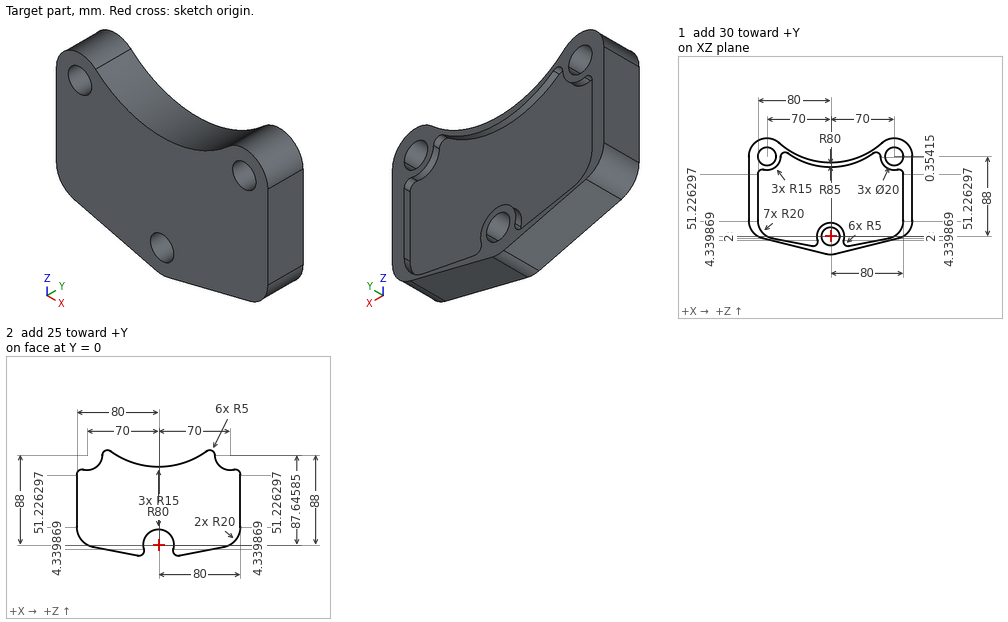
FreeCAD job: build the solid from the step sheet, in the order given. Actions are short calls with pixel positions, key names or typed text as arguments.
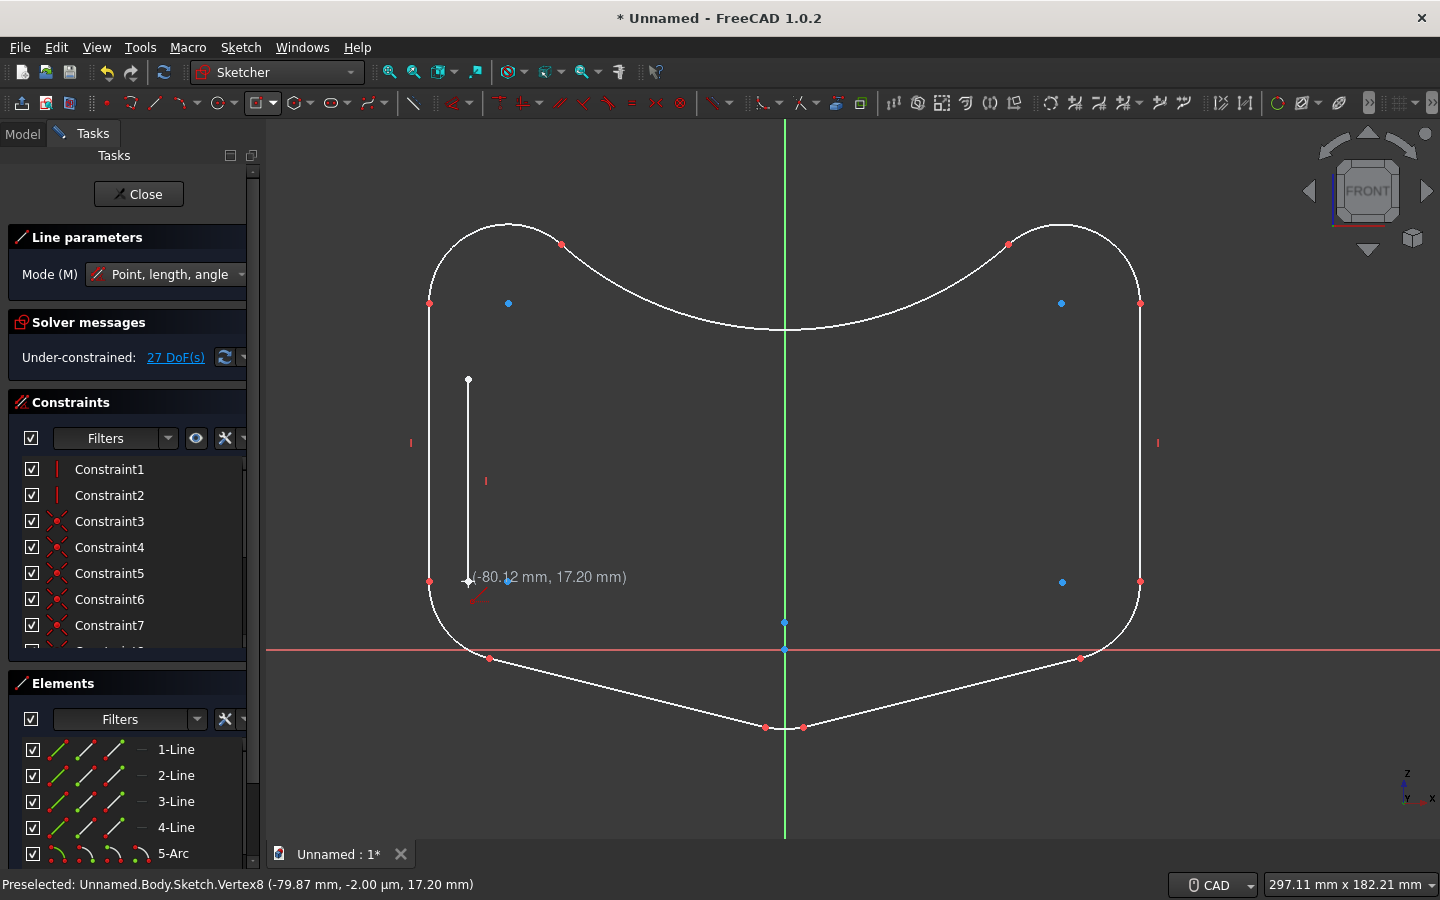
scroll(532, 659, up, 3)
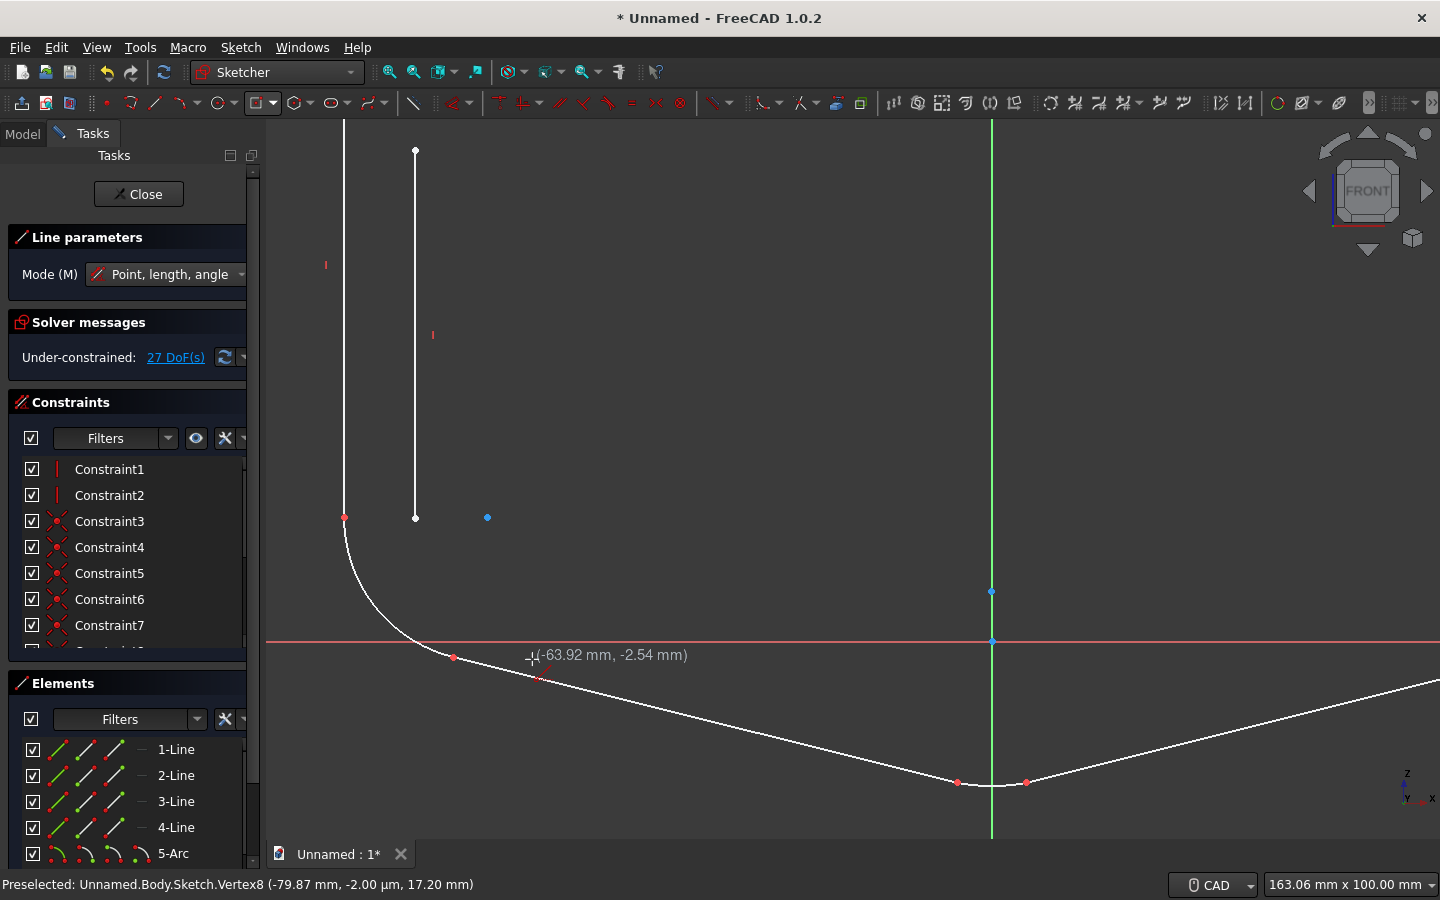
click(533, 658)
click(847, 719)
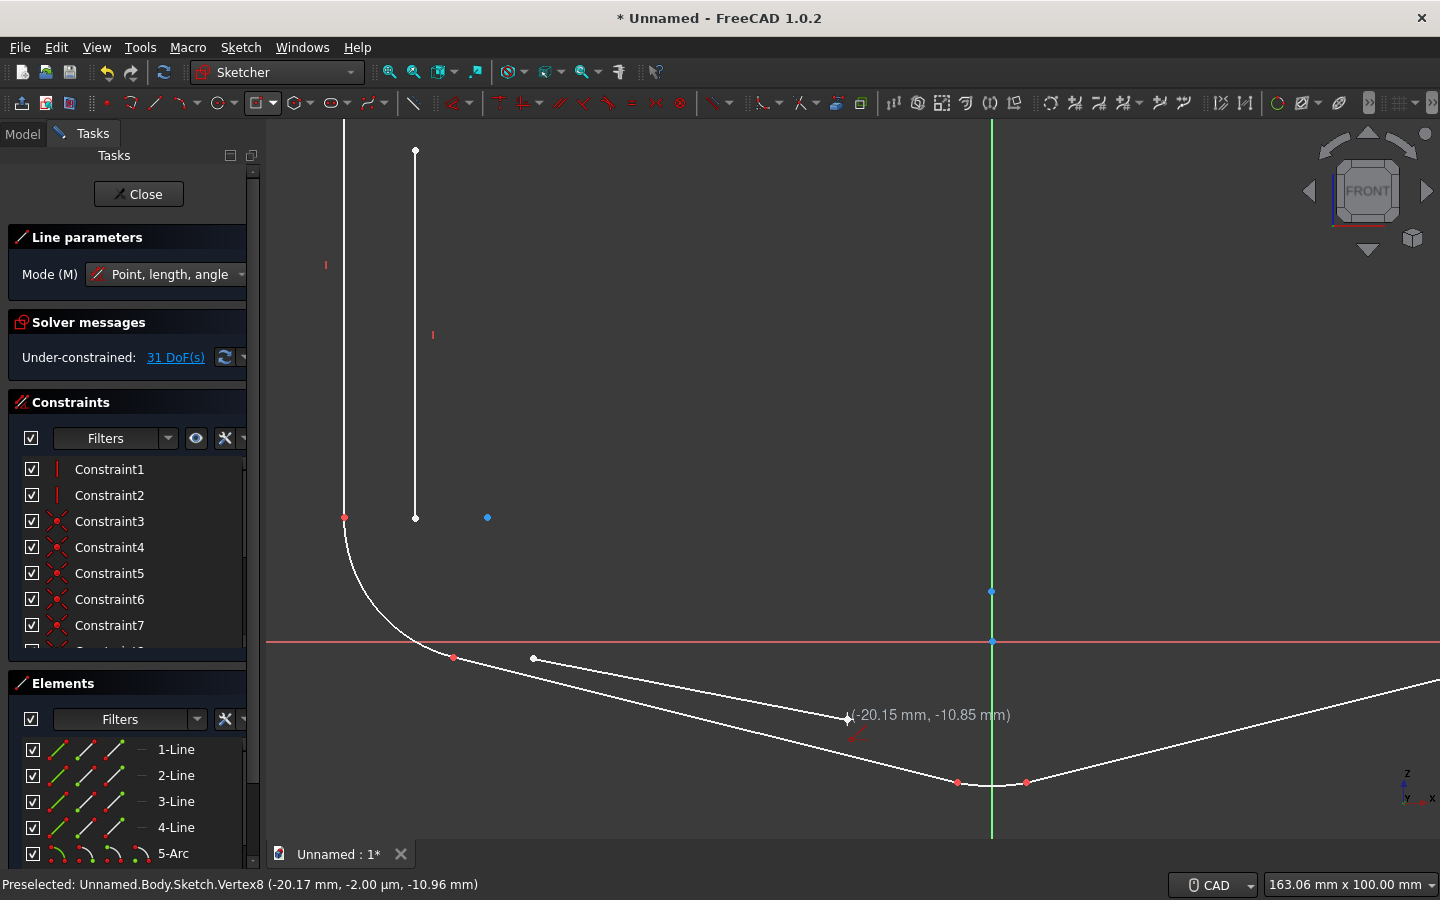
click(1137, 719)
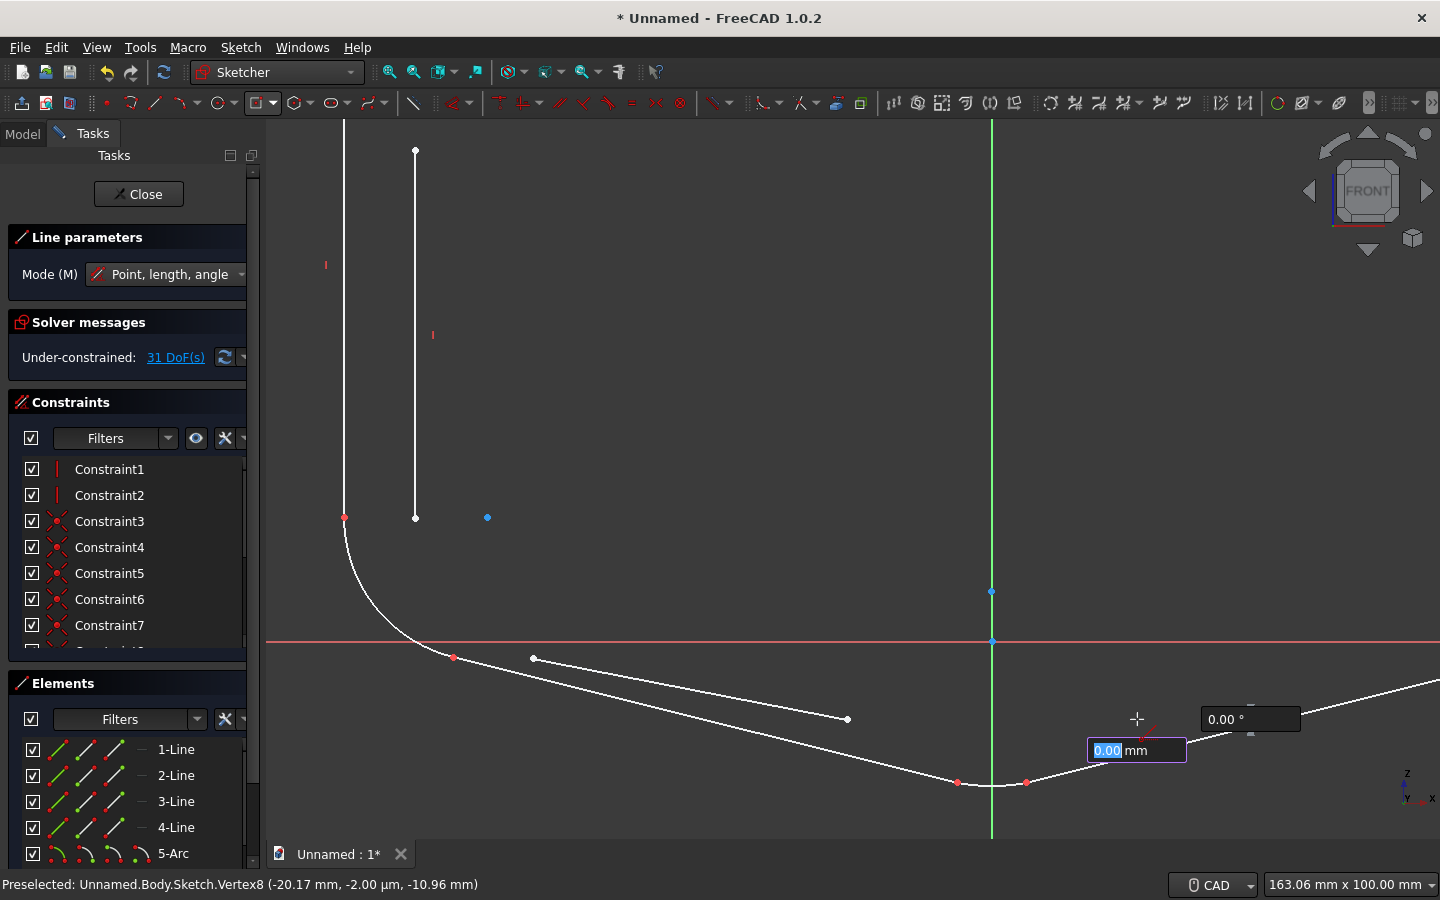
scroll(532, 659, down, 3)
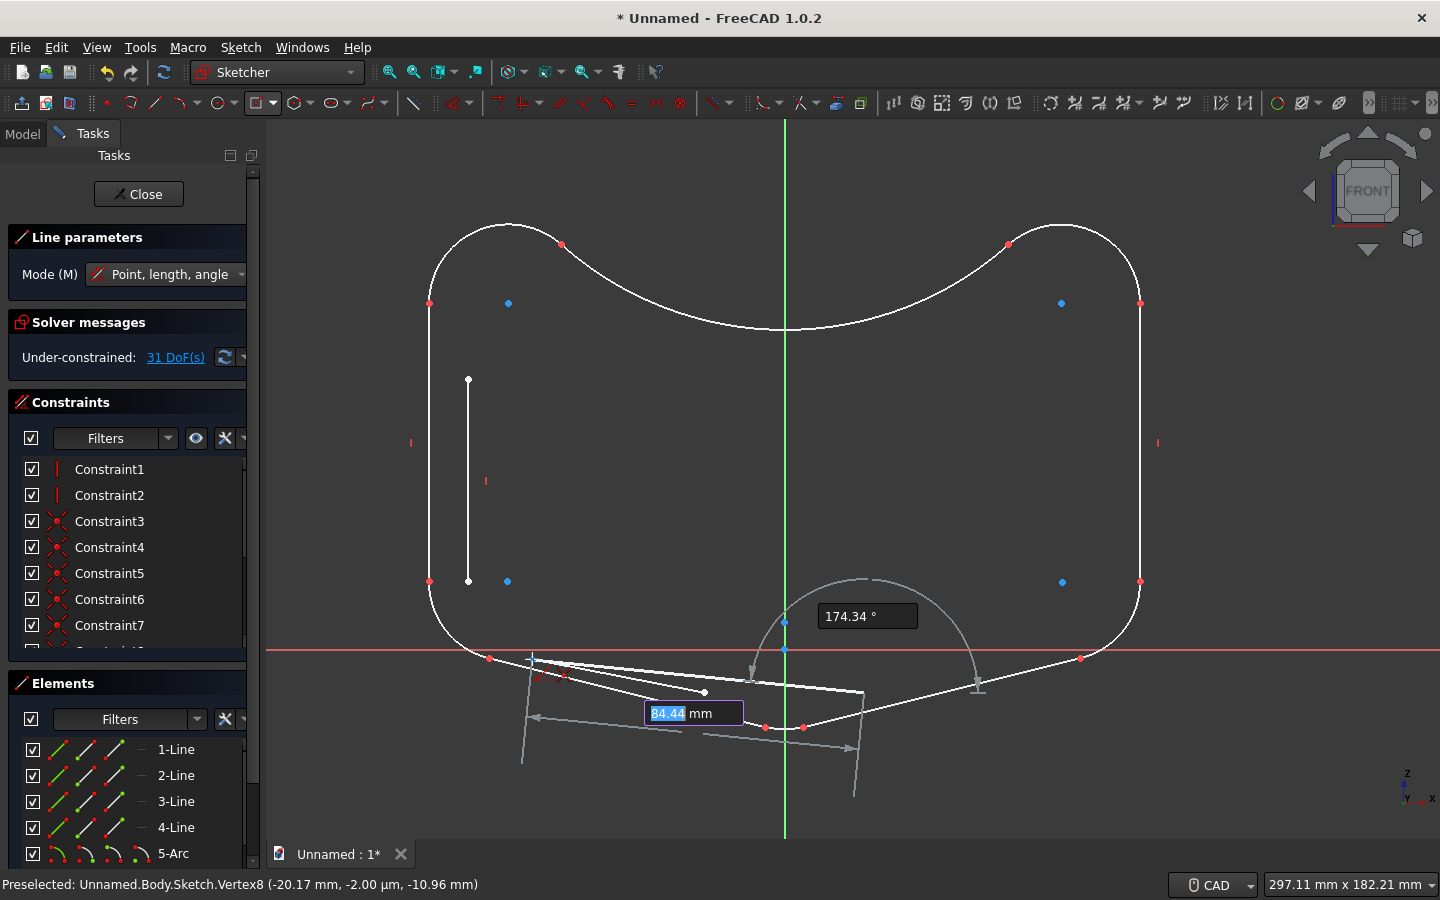
scroll(1037, 659, up, 3)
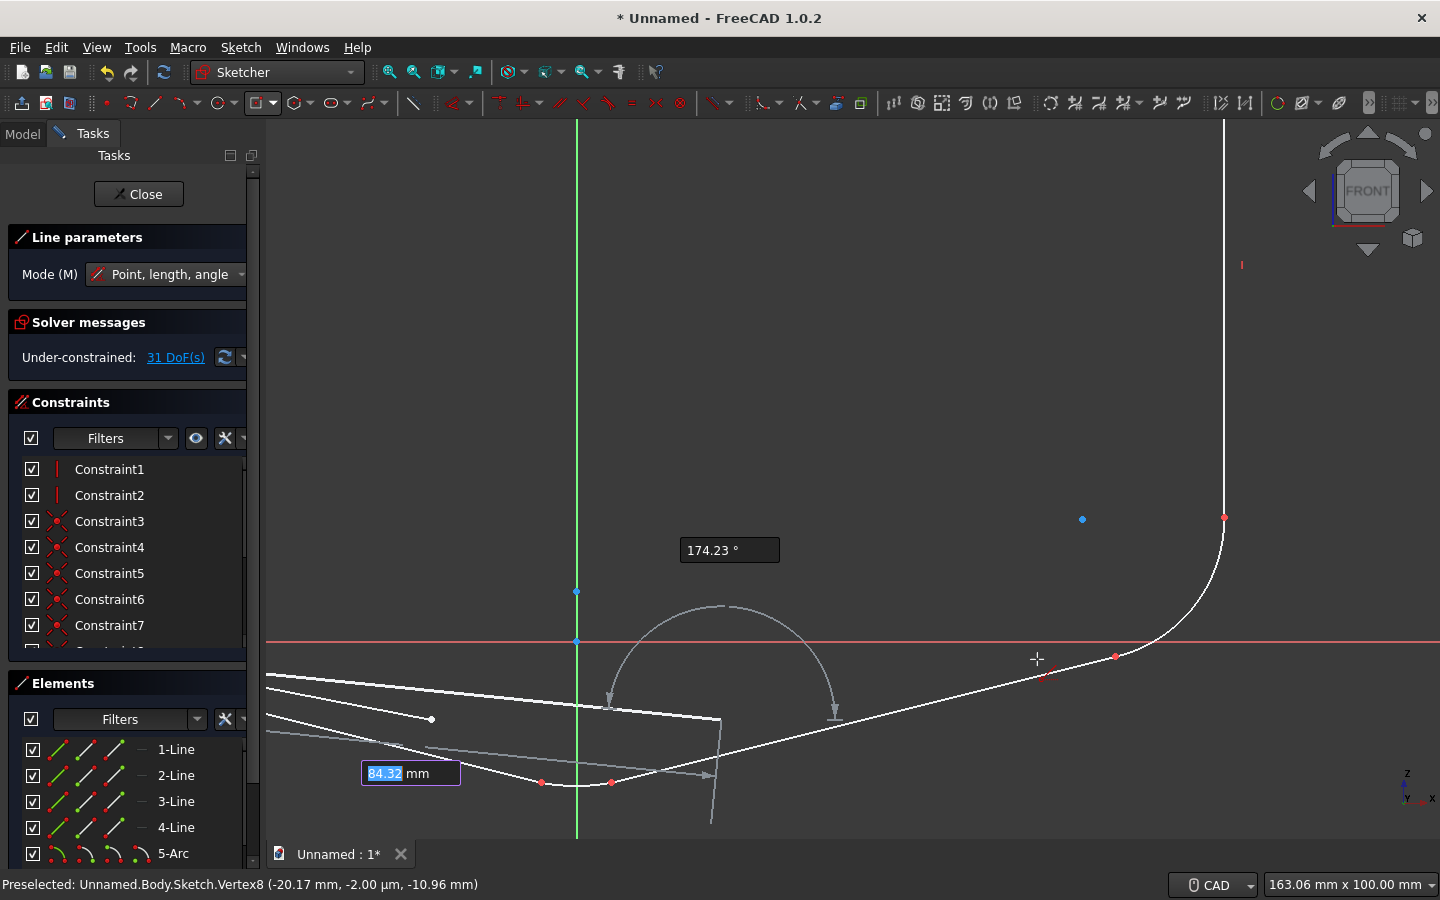
click(1036, 658)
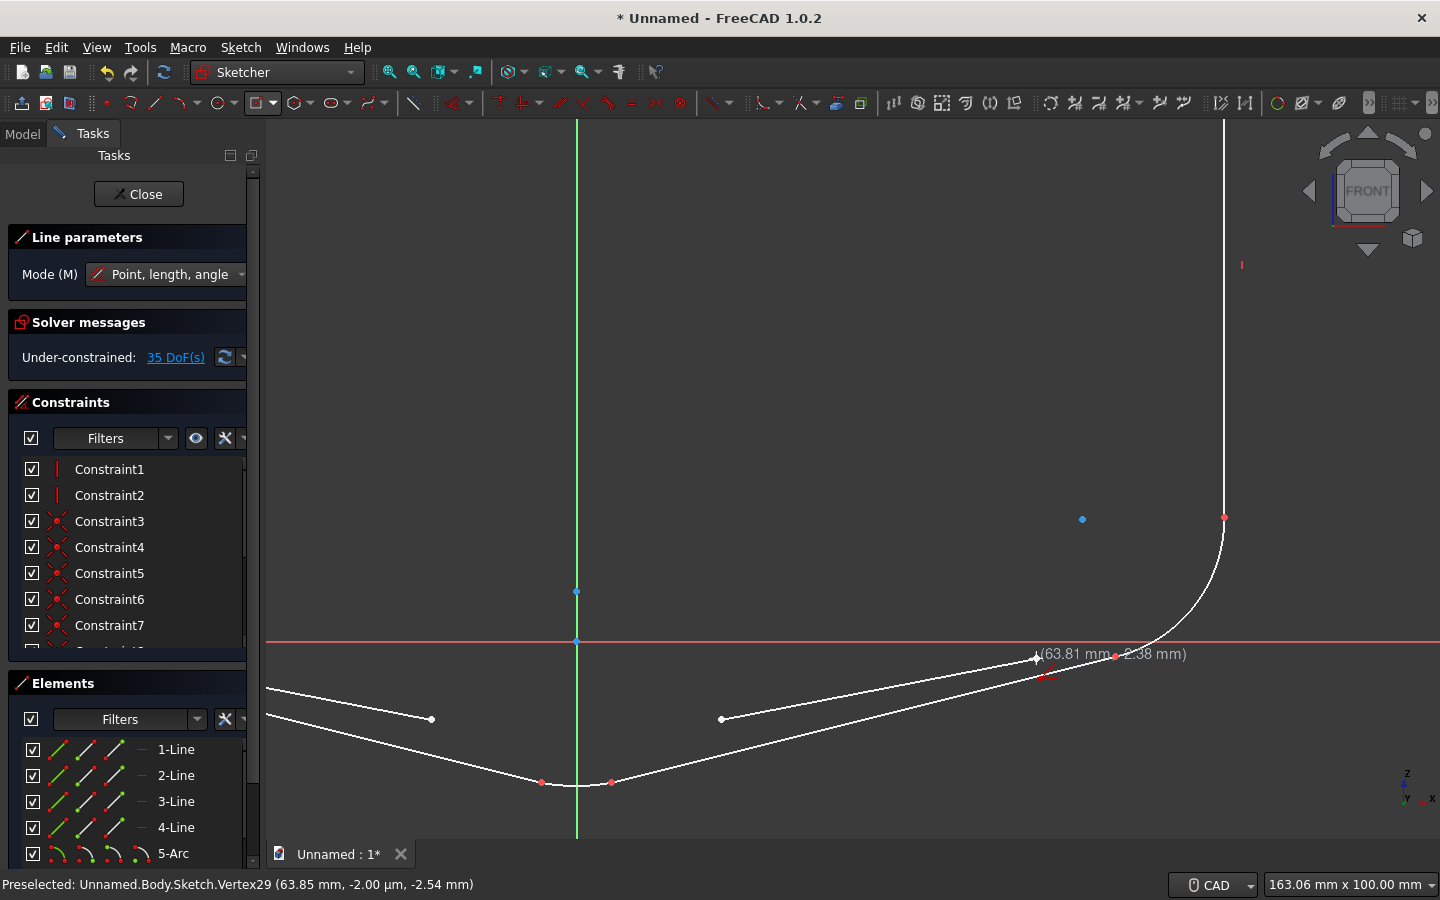
click(1153, 517)
click(1153, 148)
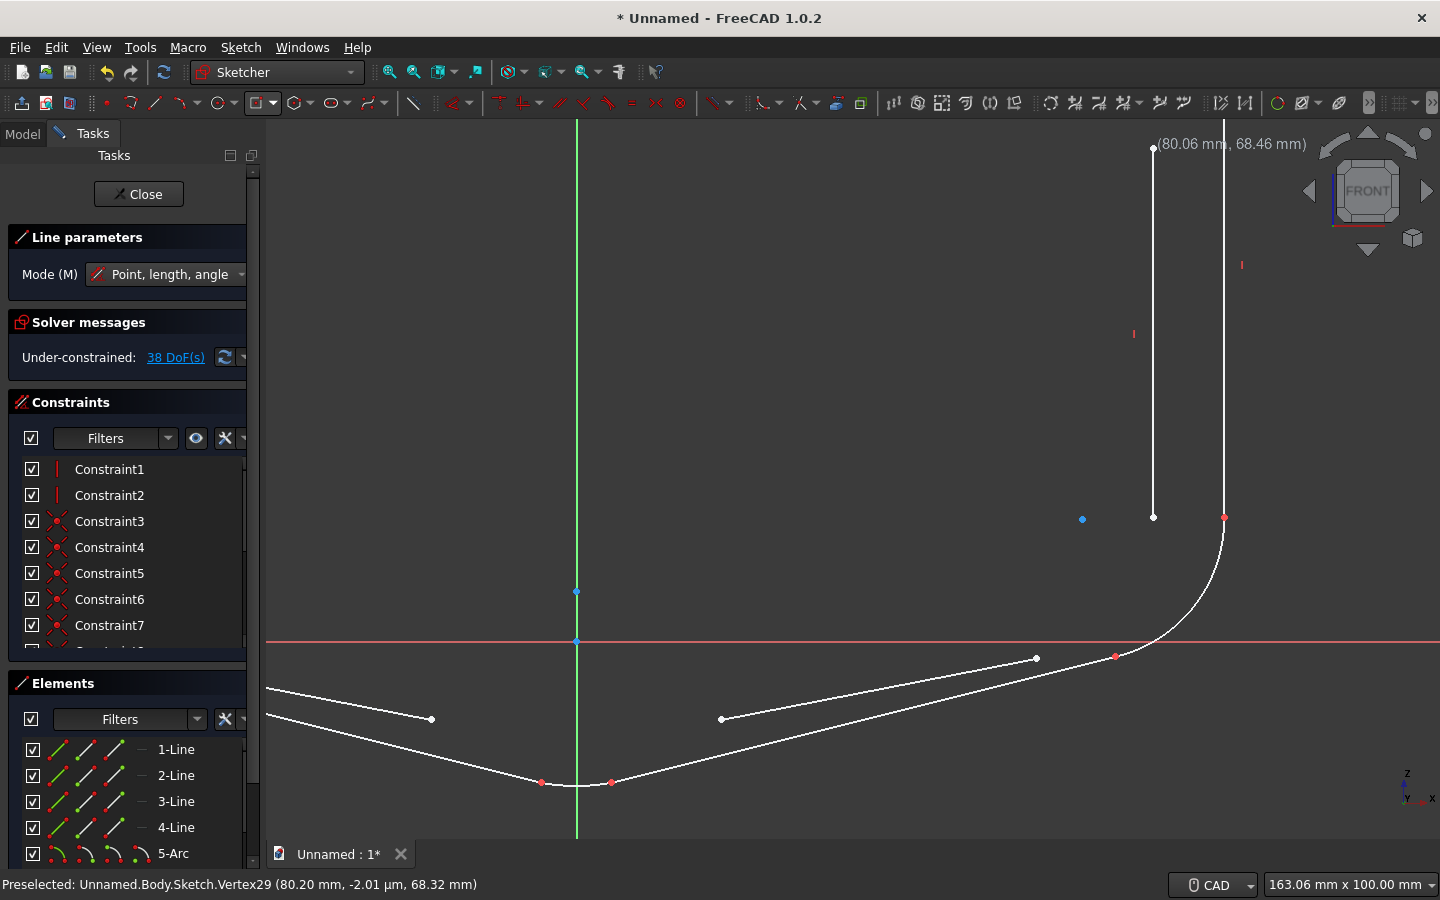
click(180, 104)